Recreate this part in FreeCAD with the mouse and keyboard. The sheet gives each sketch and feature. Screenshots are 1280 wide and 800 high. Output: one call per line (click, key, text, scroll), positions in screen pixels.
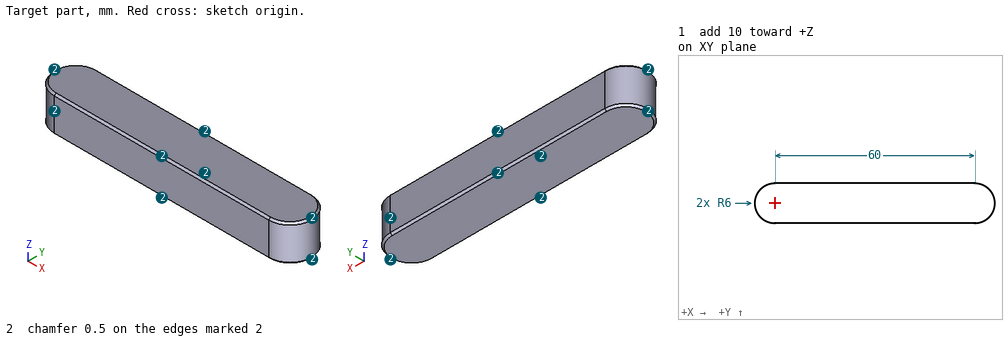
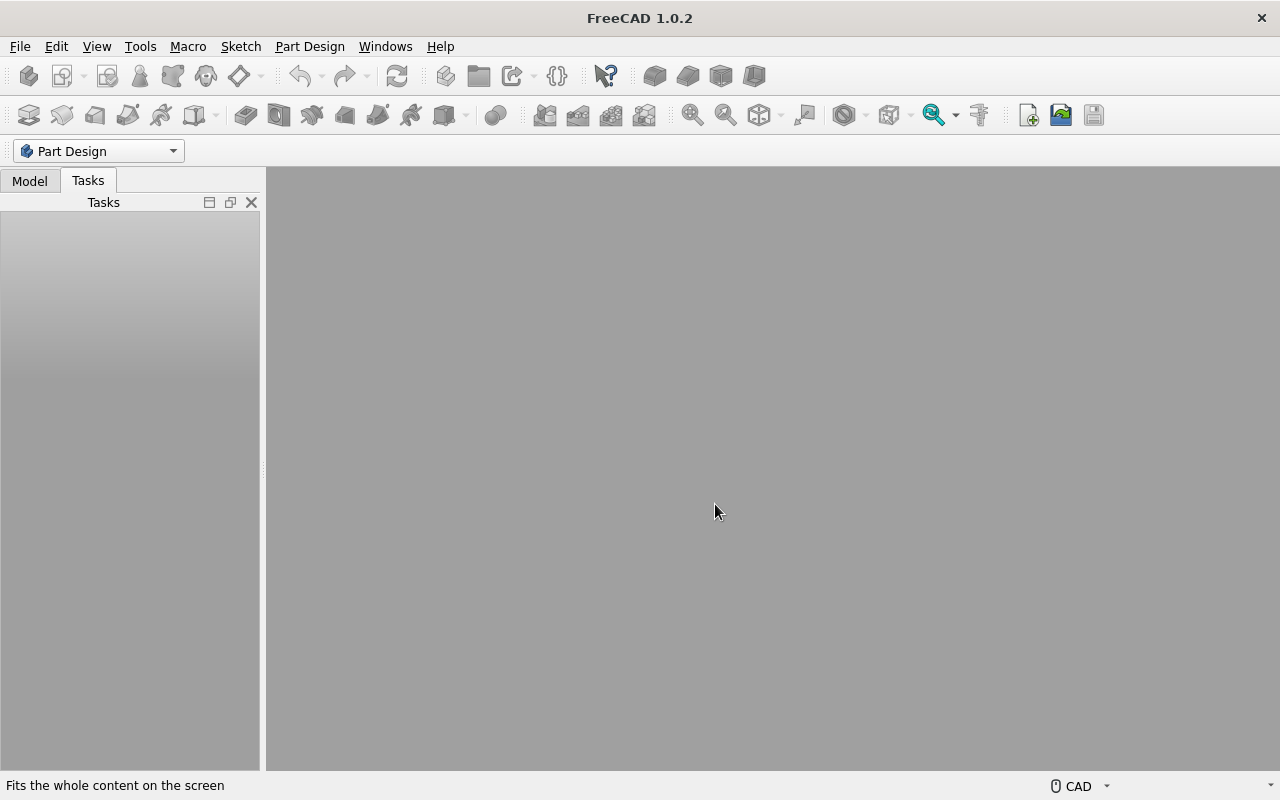
click(1028, 116)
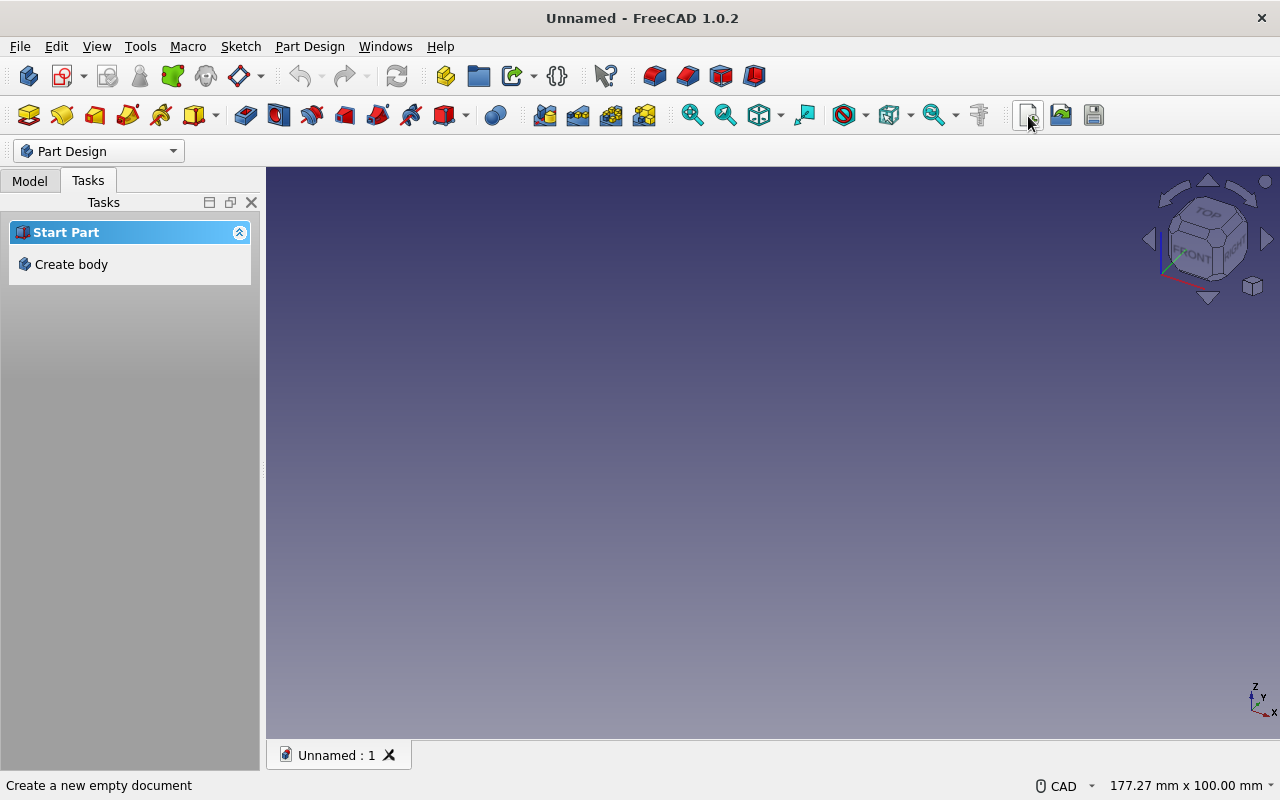
click(62, 76)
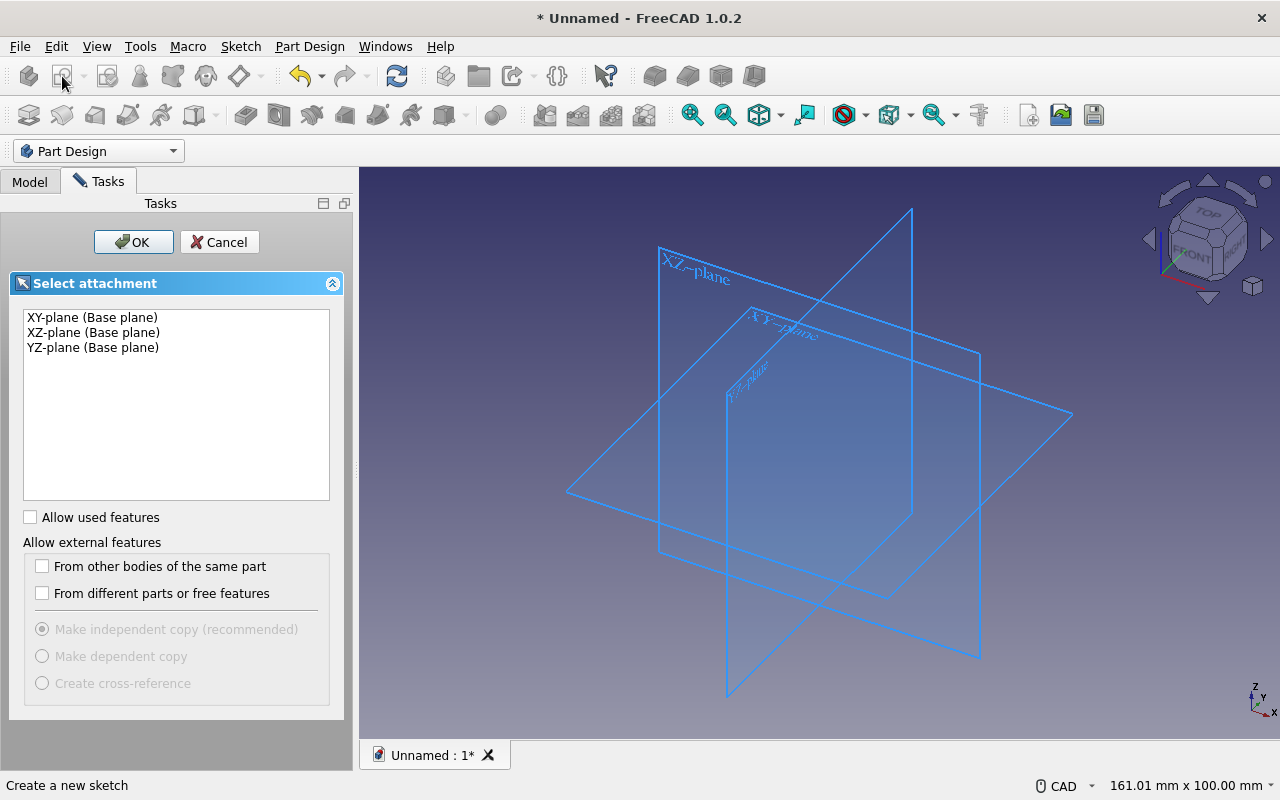
click(84, 318)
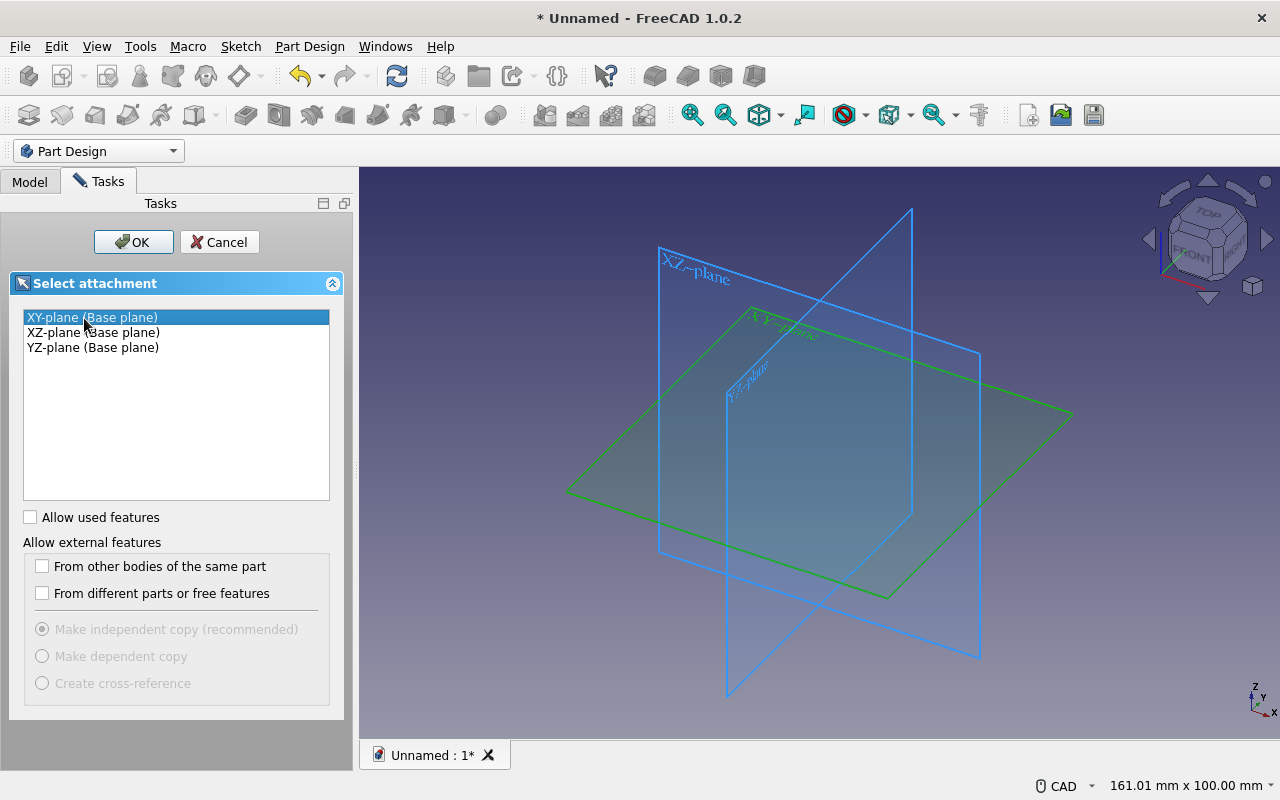
click(134, 242)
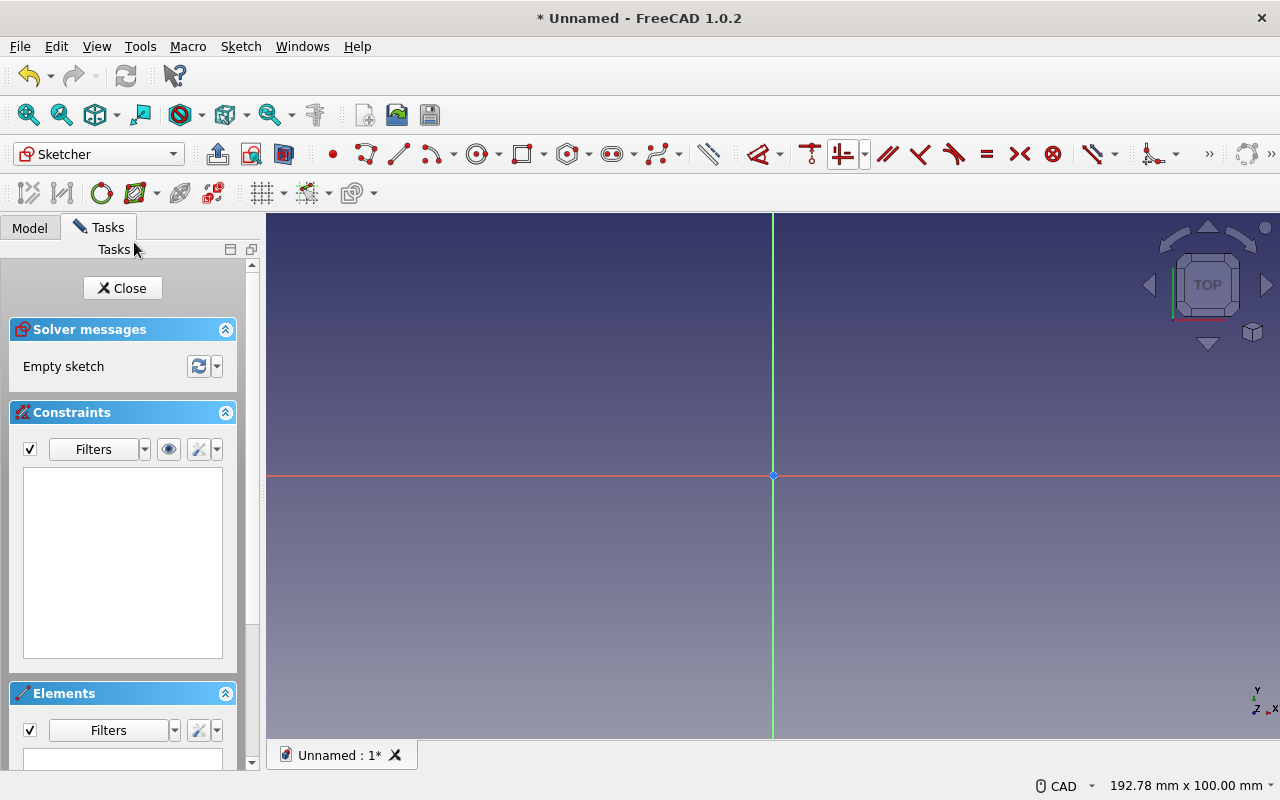
scroll(294, 476, down, 1)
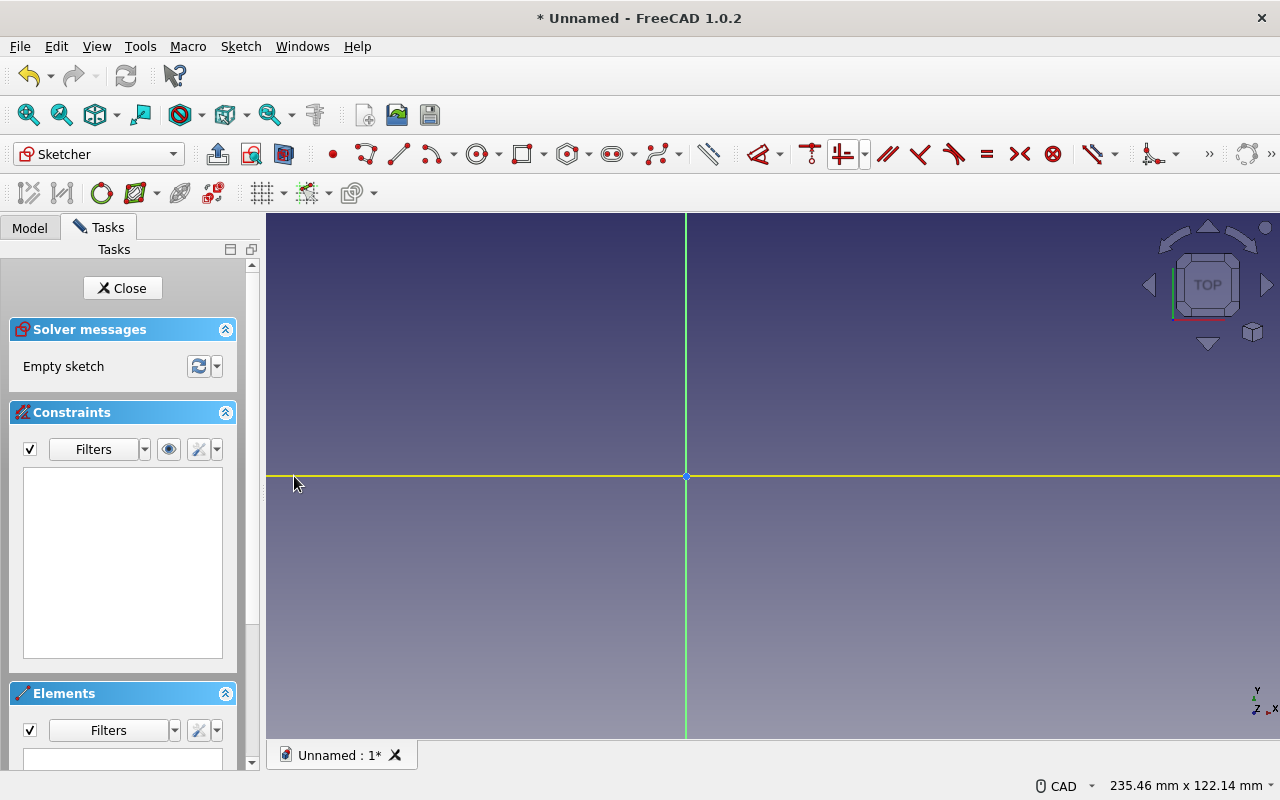
scroll(950, 476, up, 3)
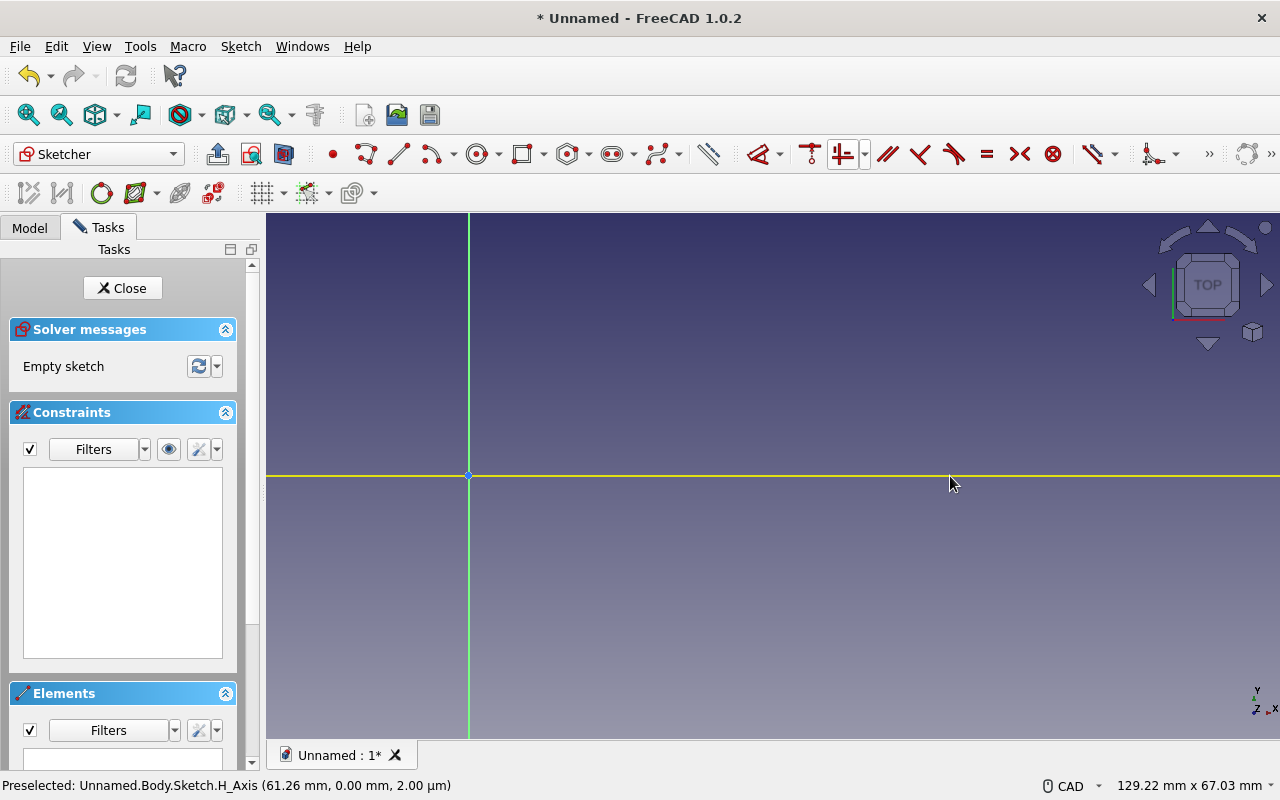
click(612, 154)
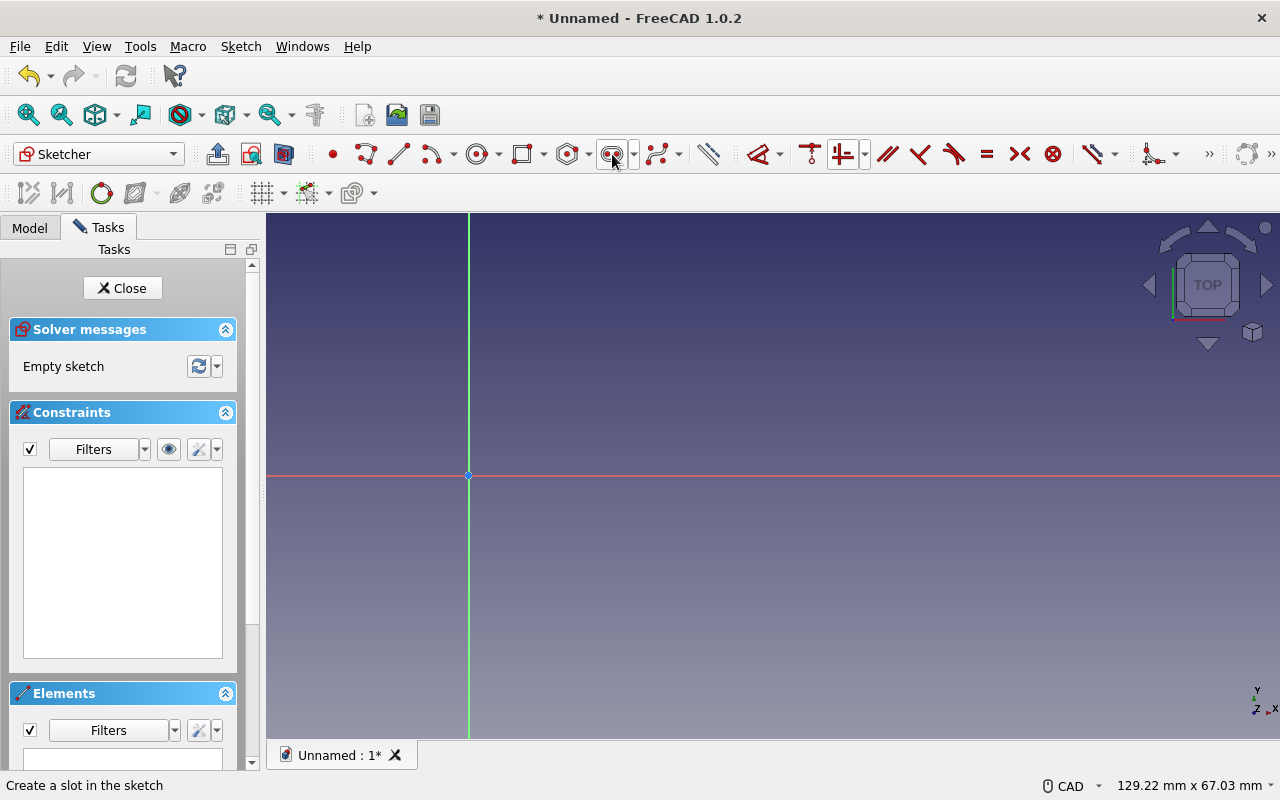
click(469, 476)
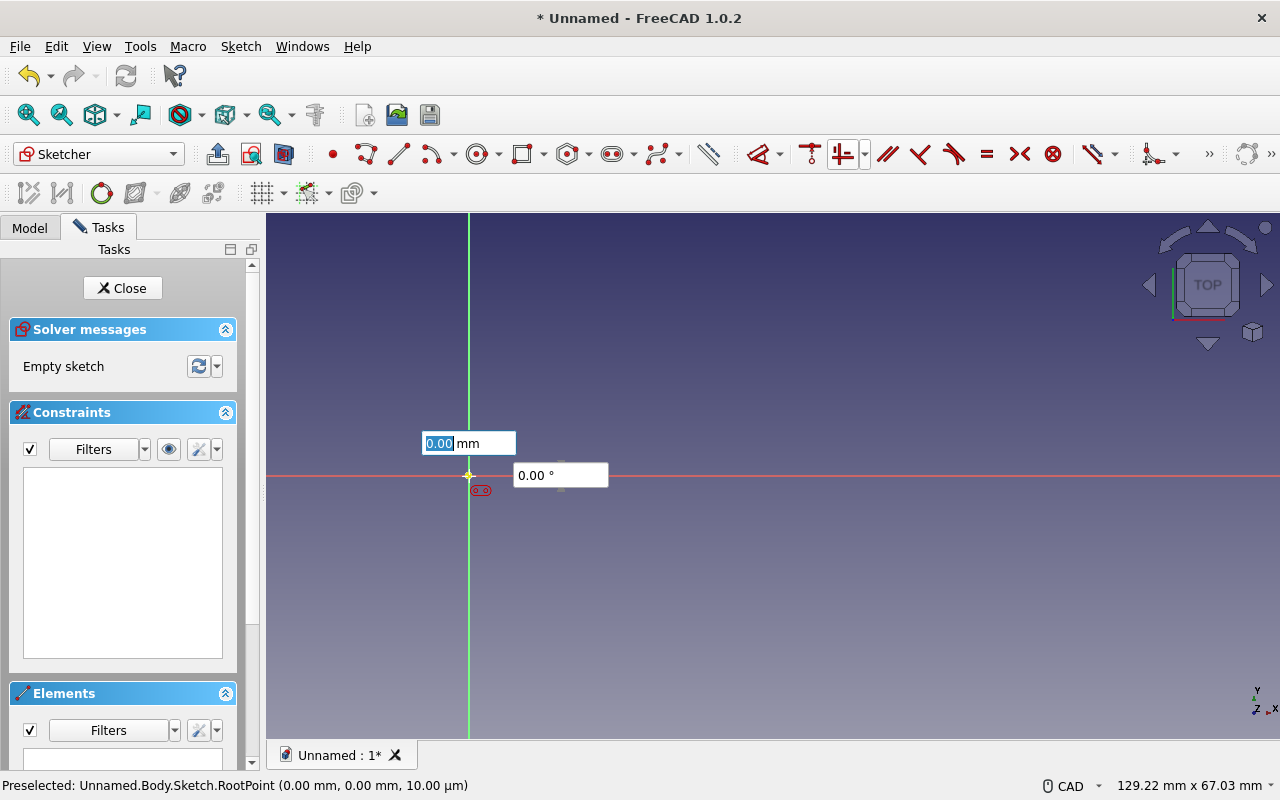
click(940, 467)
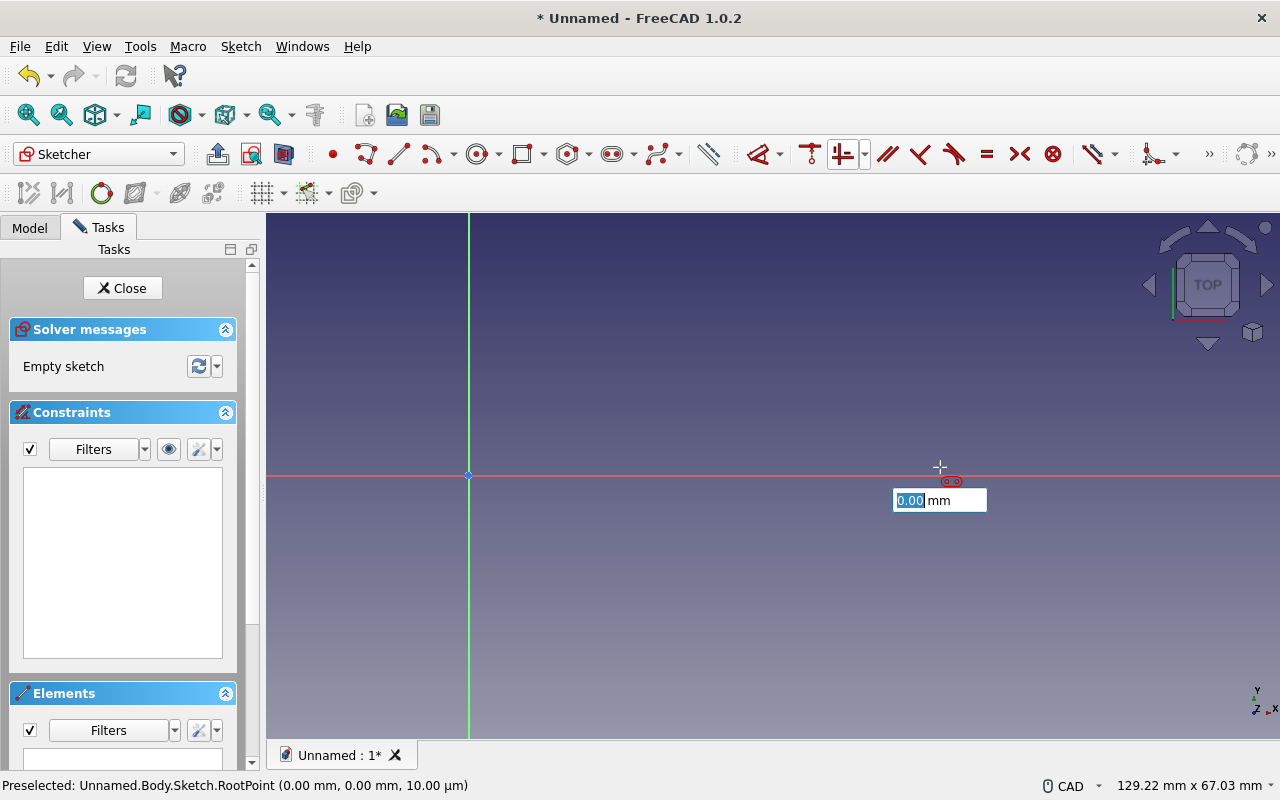
click(704, 429)
key(Escape)